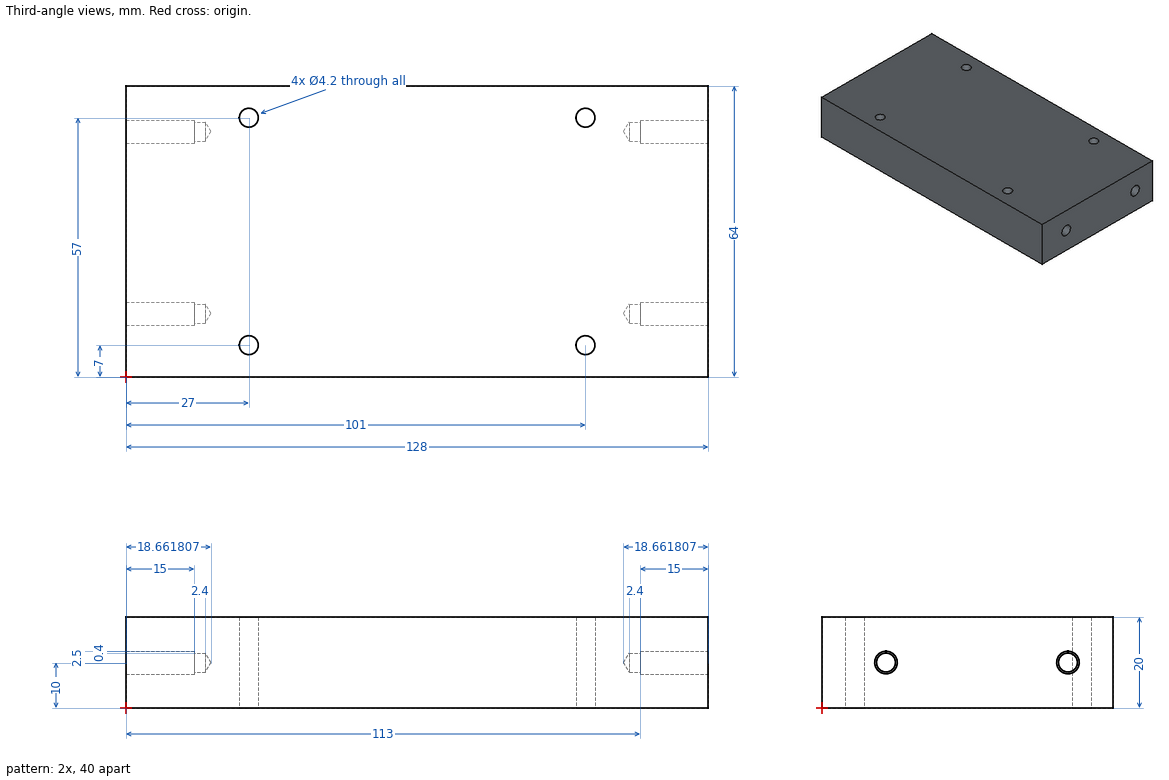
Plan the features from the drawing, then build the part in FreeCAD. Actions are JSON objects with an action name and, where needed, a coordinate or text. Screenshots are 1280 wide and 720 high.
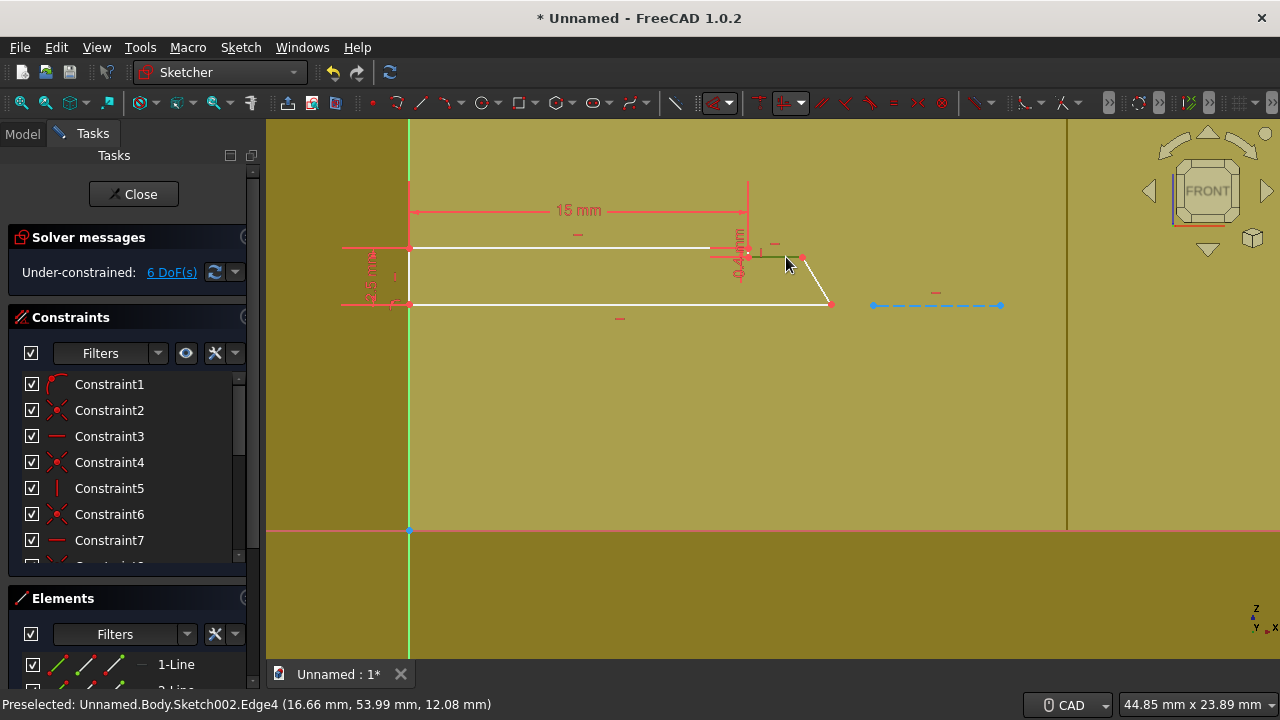
{"action": "left_click", "coordinate": [732, 104]}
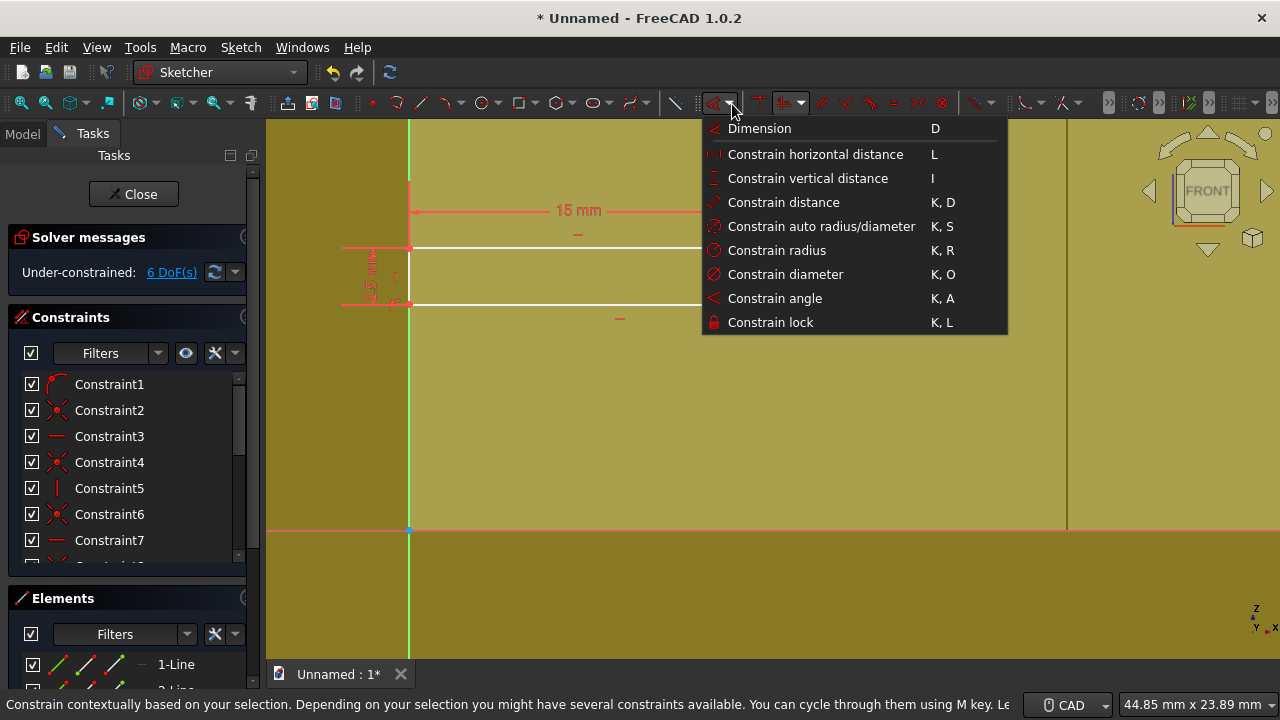
{"action": "left_click", "coordinate": [855, 154]}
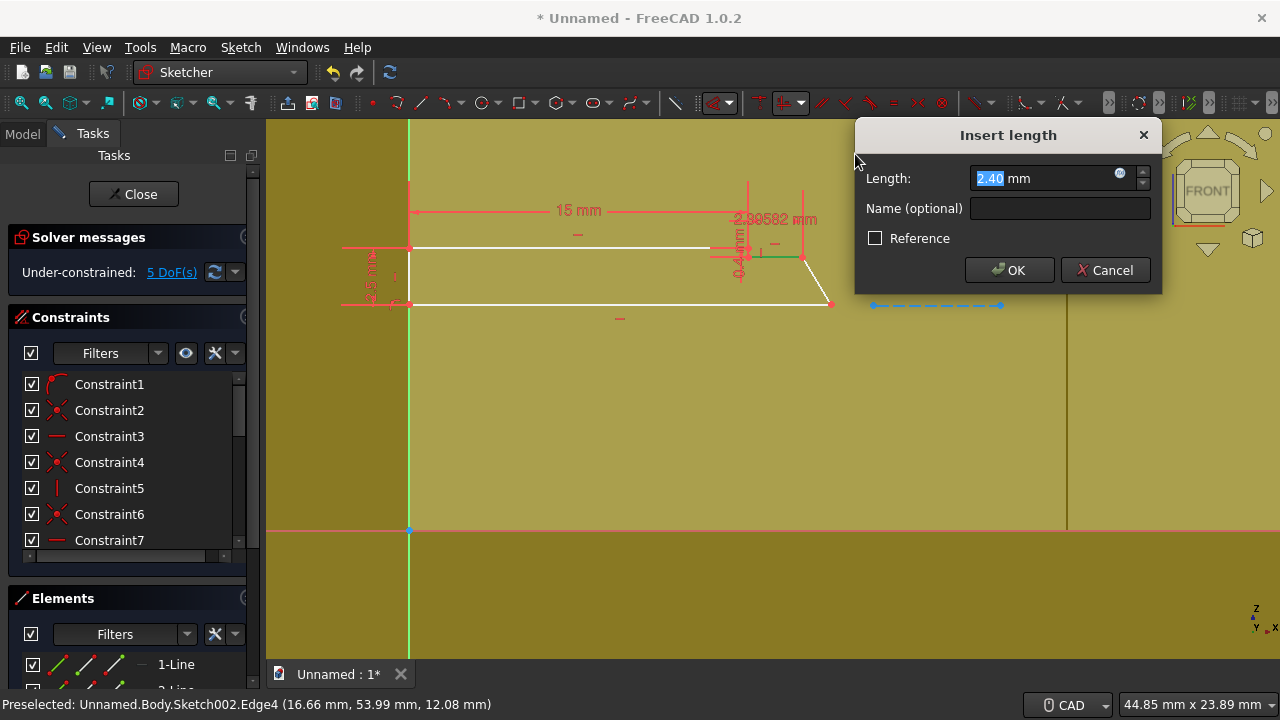
{"action": "type", "text": "2.4"}
{"action": "key", "text": "Return"}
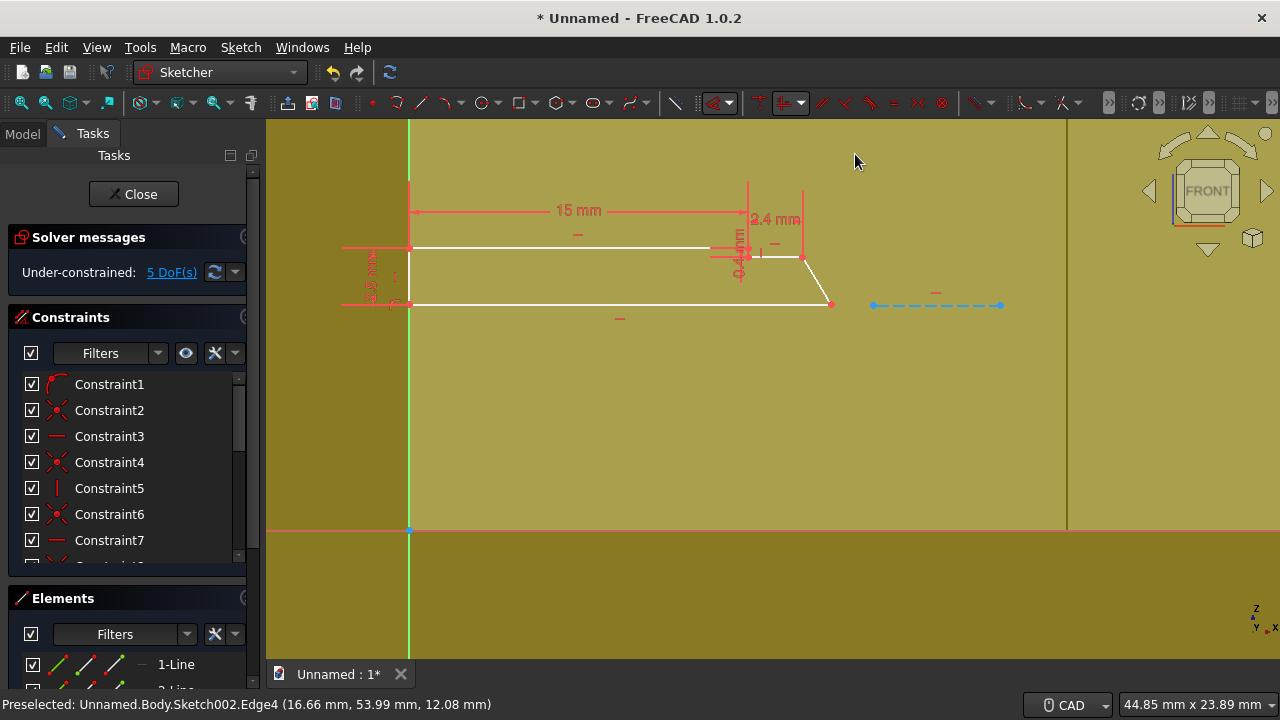
{"action": "left_click", "coordinate": [409, 305]}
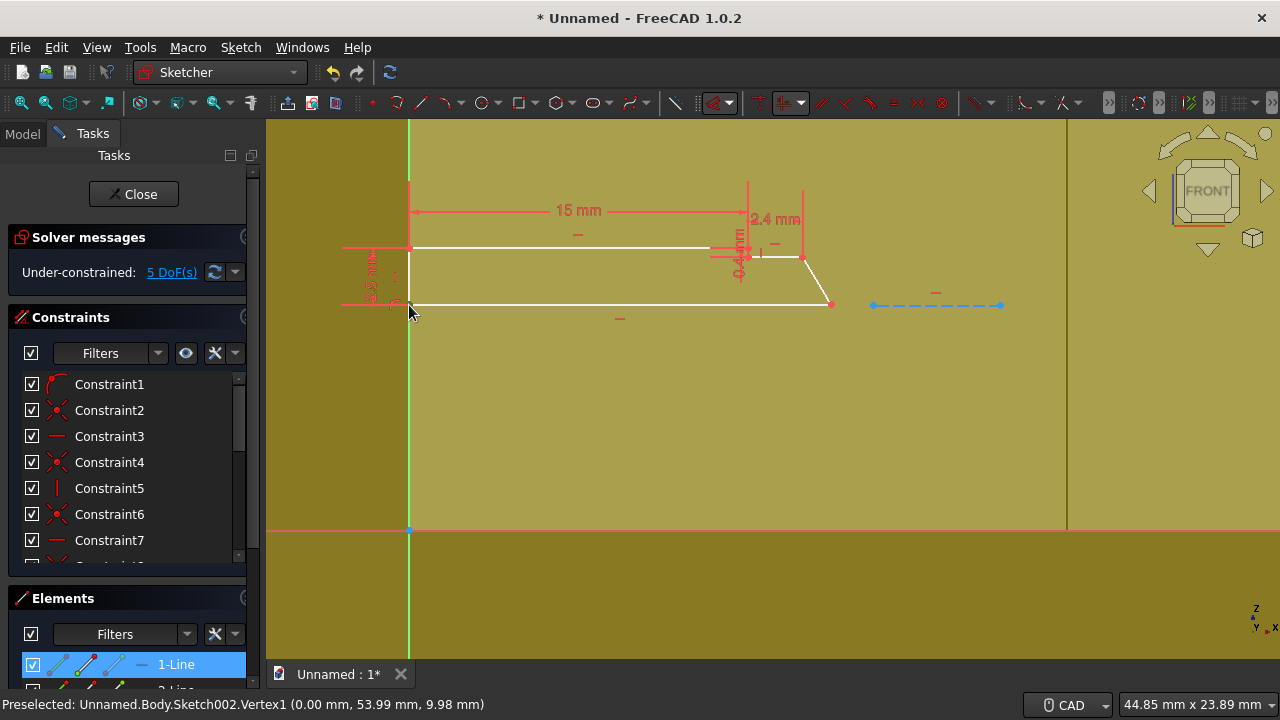
{"action": "left_click", "coordinate": [732, 104]}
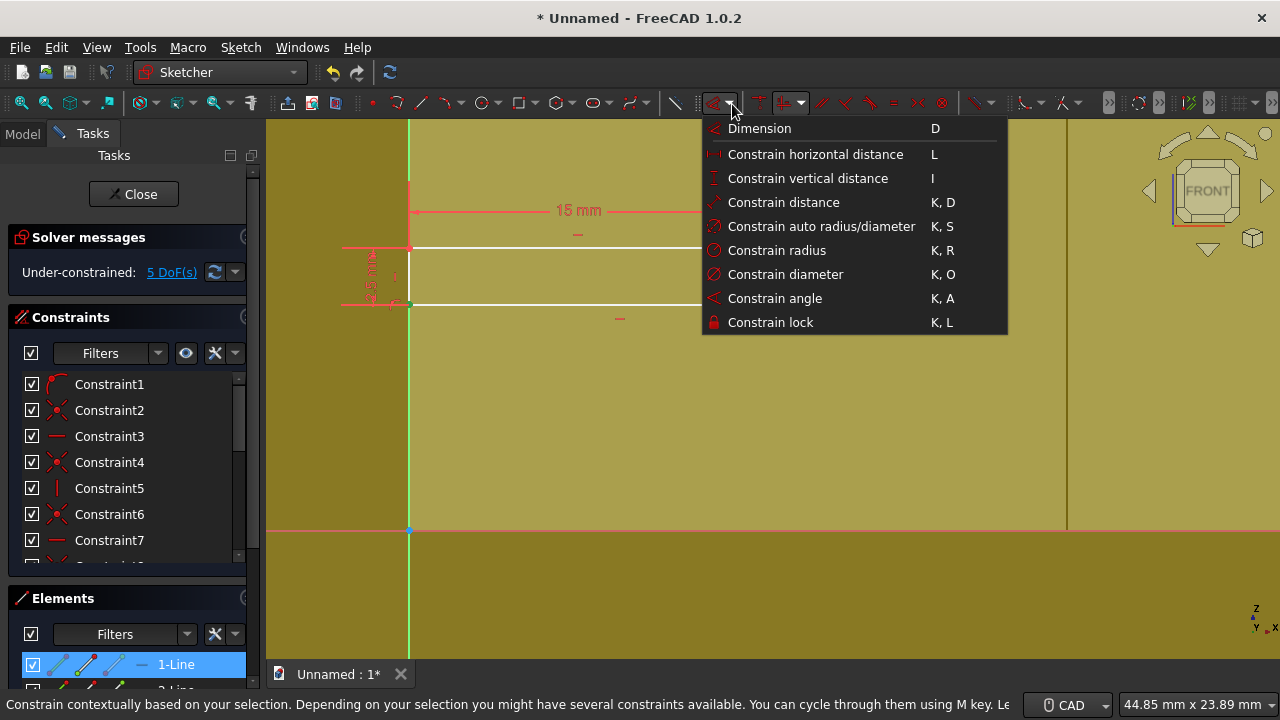
{"action": "left_click", "coordinate": [855, 178]}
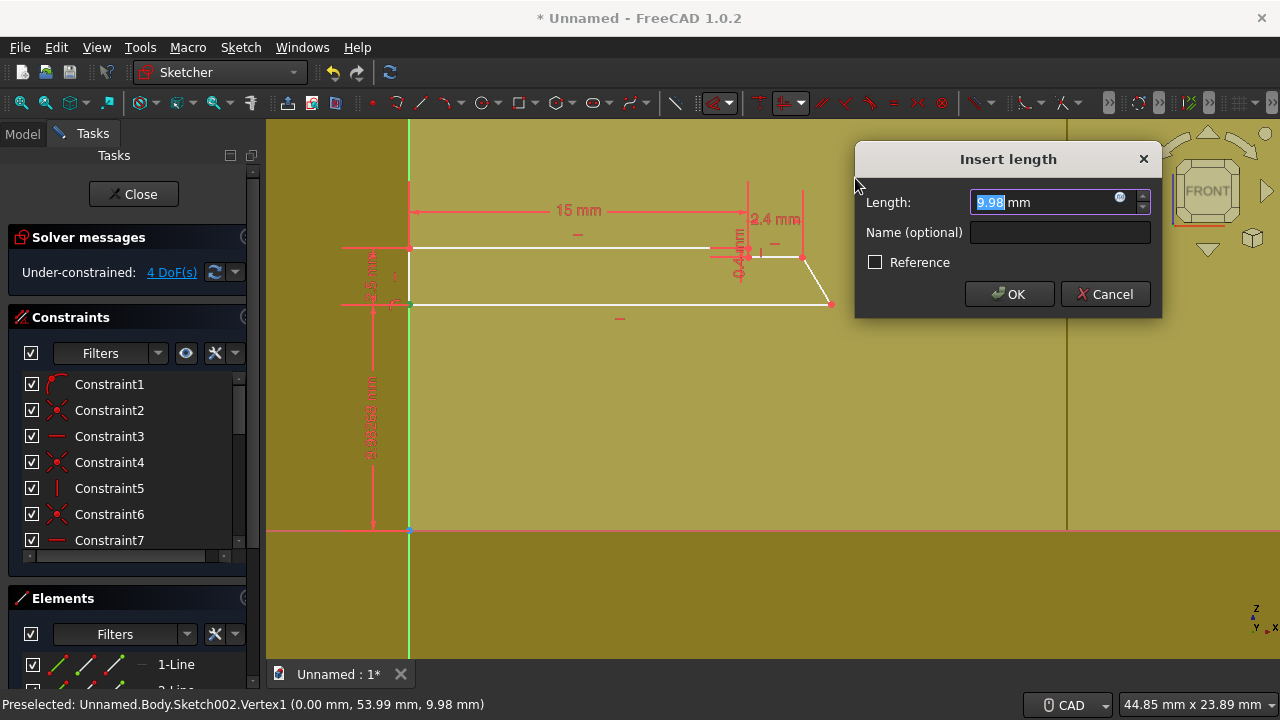
{"action": "type", "text": "10"}
{"action": "key", "text": "Return"}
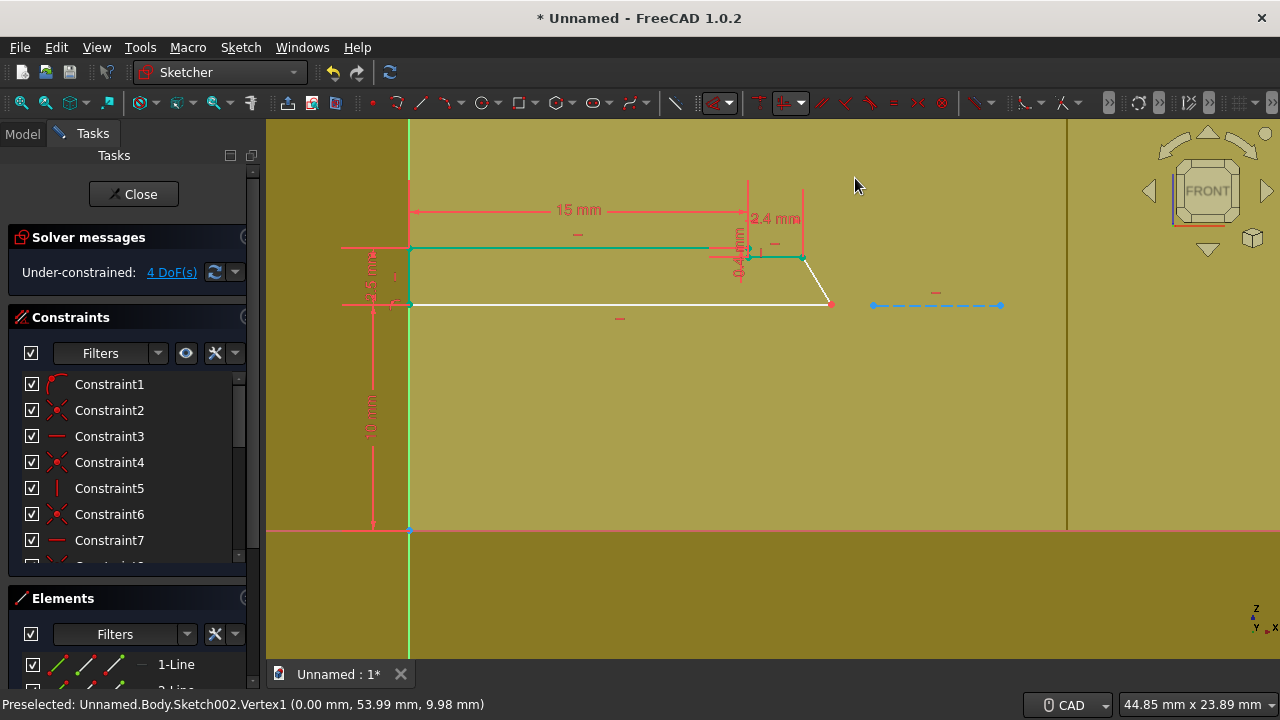
{"action": "left_click", "coordinate": [873, 306]}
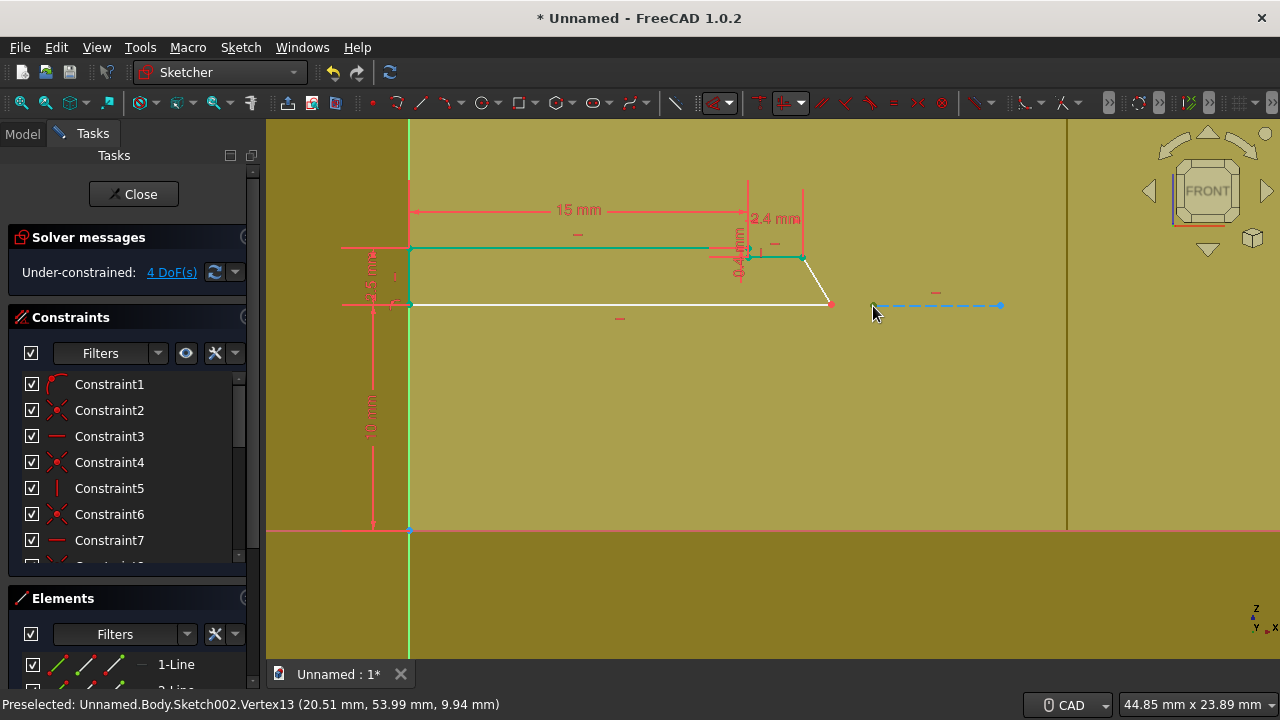
{"action": "key", "text": "i"}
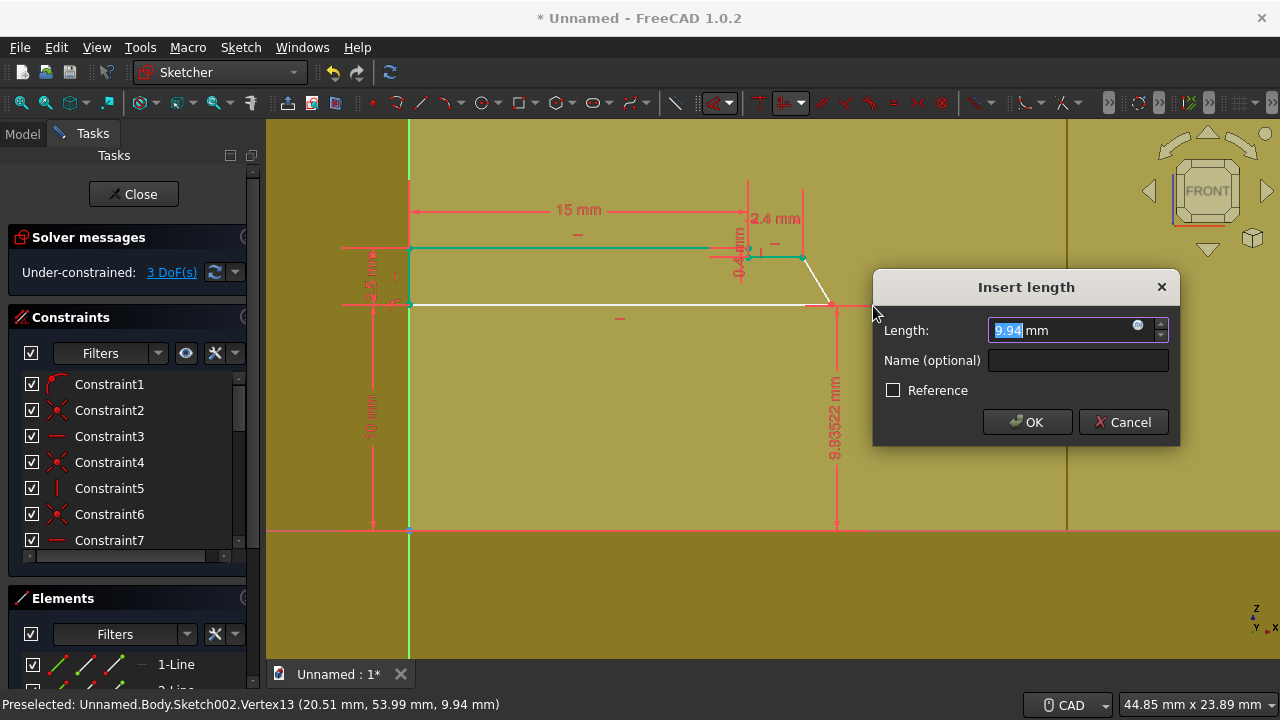
{"action": "type", "text": "10"}
{"action": "key", "text": "Return"}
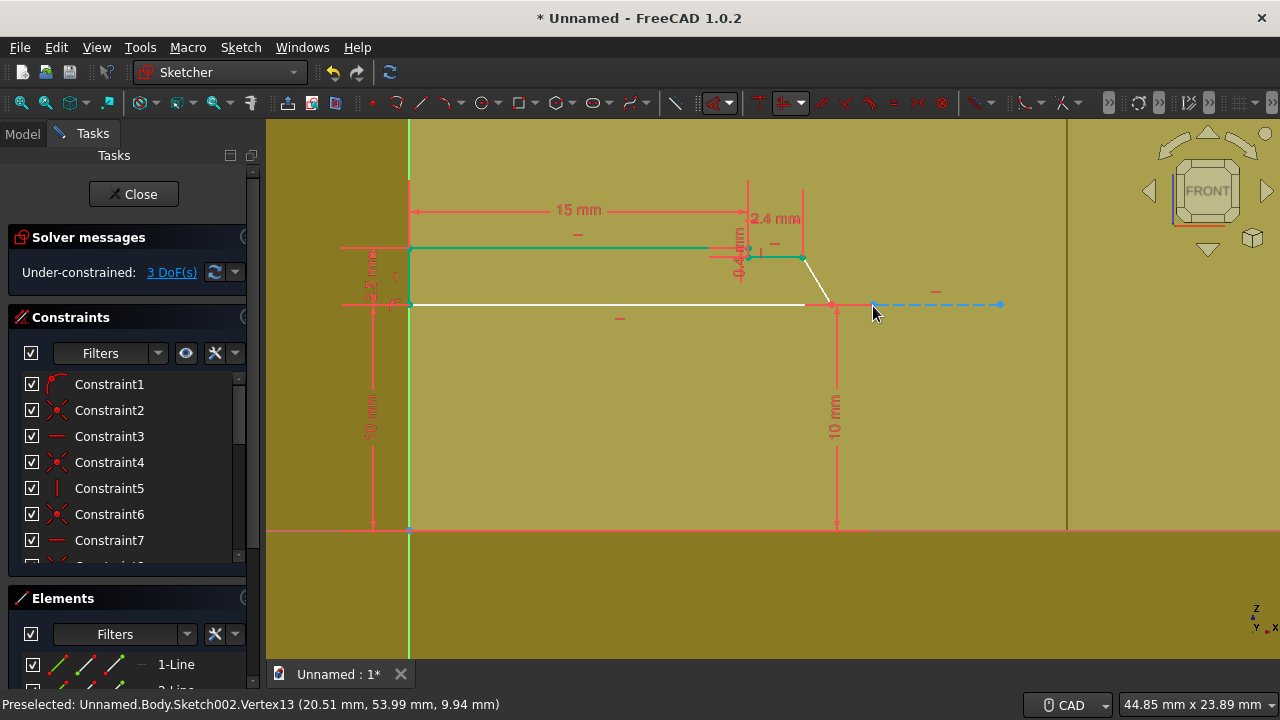
{"action": "left_click", "coordinate": [705, 305]}